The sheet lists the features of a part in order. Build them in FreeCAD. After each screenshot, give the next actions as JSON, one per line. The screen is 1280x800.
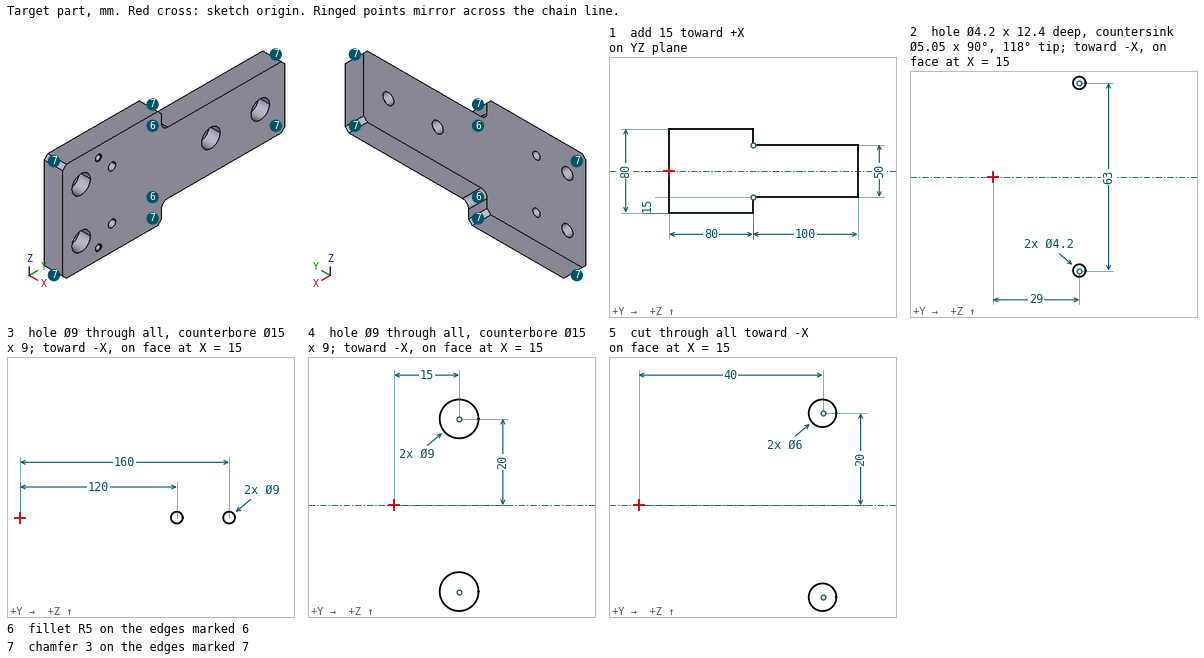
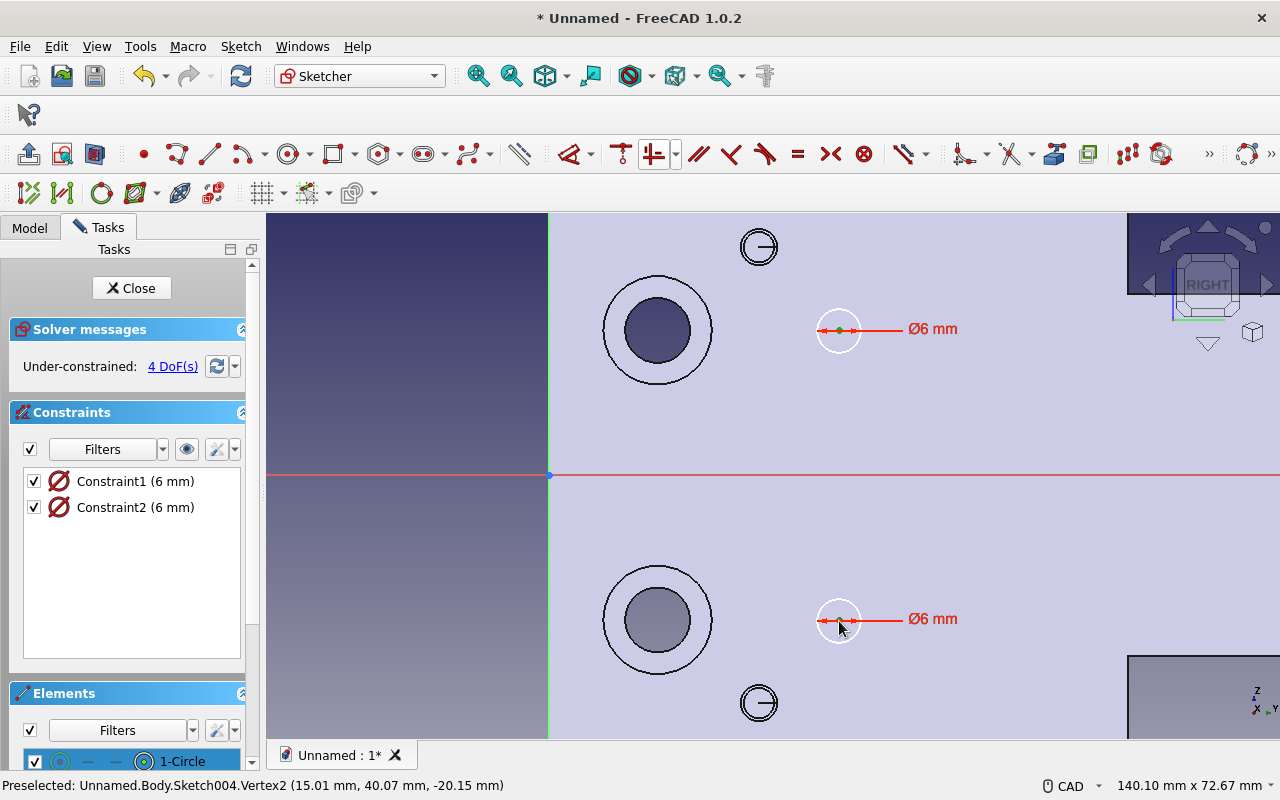
{"action": "left_click", "coordinate": [353, 475]}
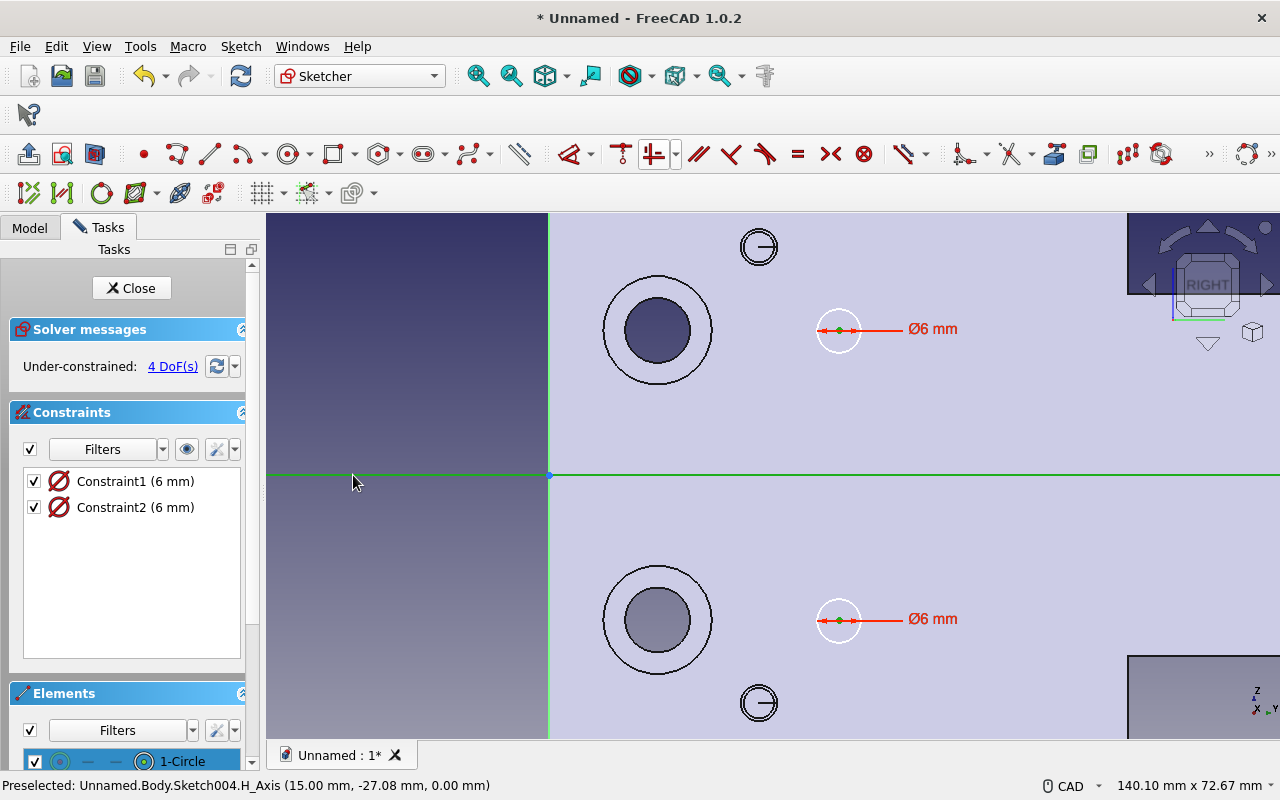
{"action": "left_click", "coordinate": [831, 154]}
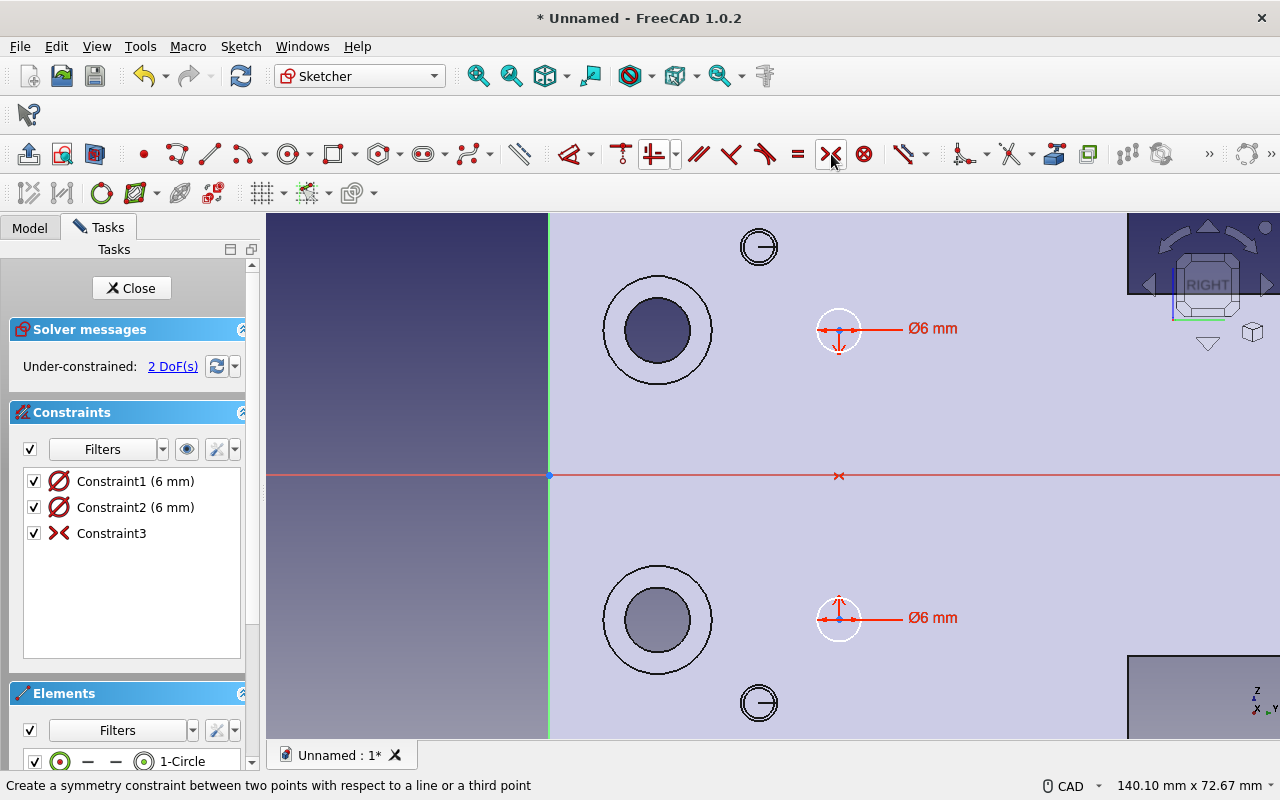
{"action": "key", "text": "d"}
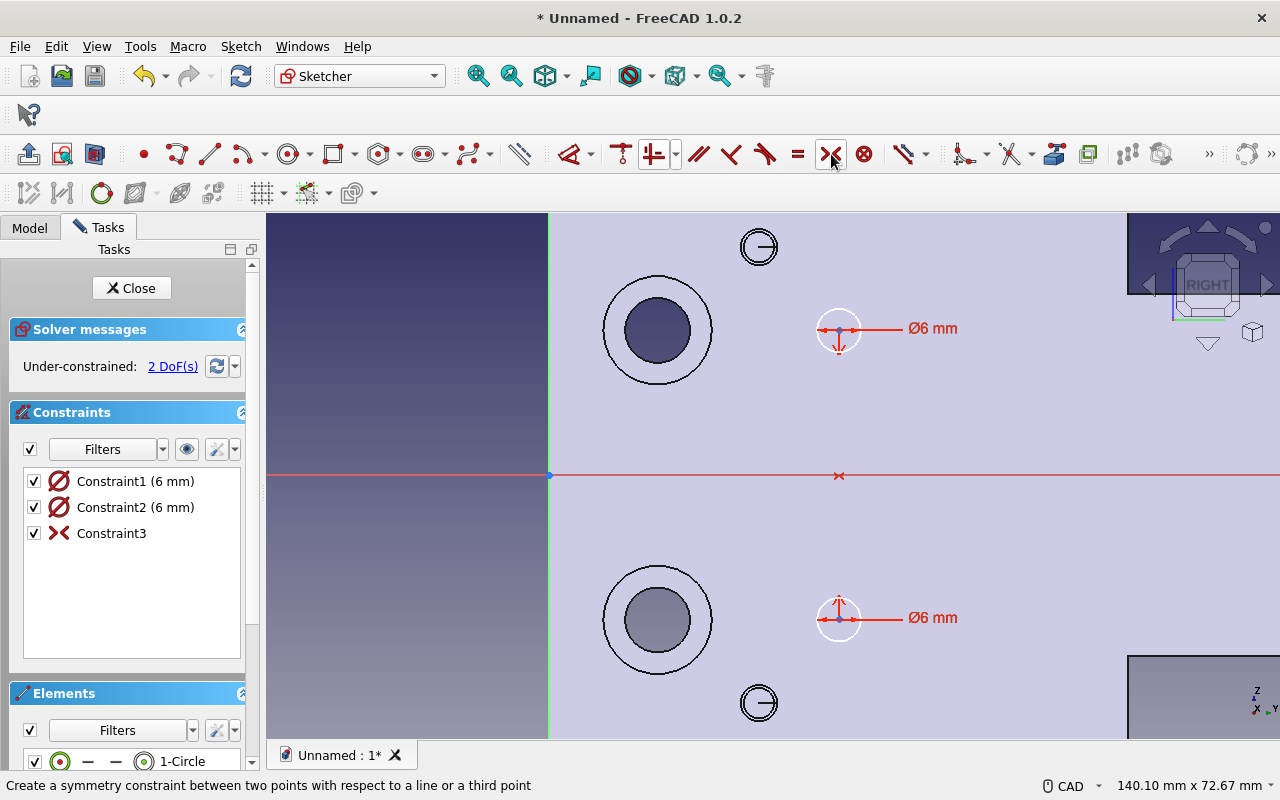
{"action": "left_click", "coordinate": [839, 330]}
{"action": "left_click", "coordinate": [694, 296]}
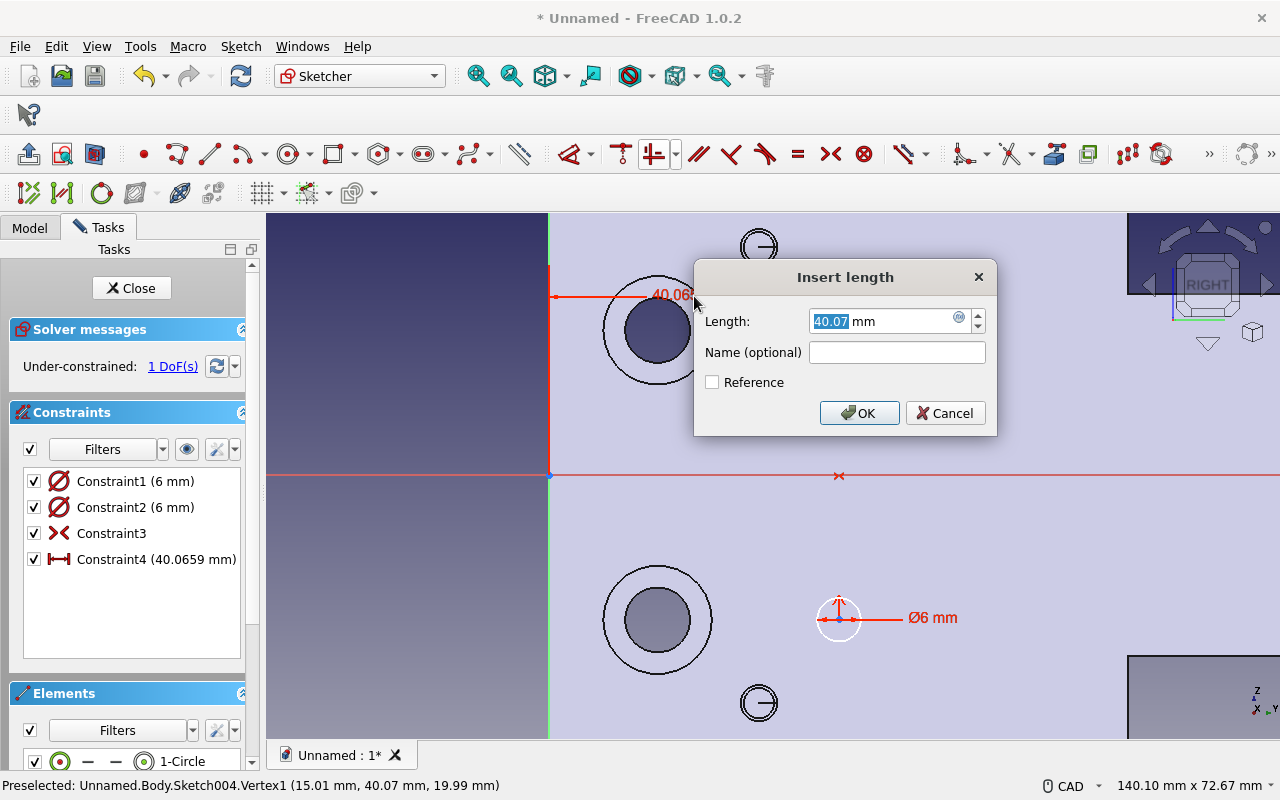
{"action": "type", "text": "40"}
{"action": "key", "text": "Return"}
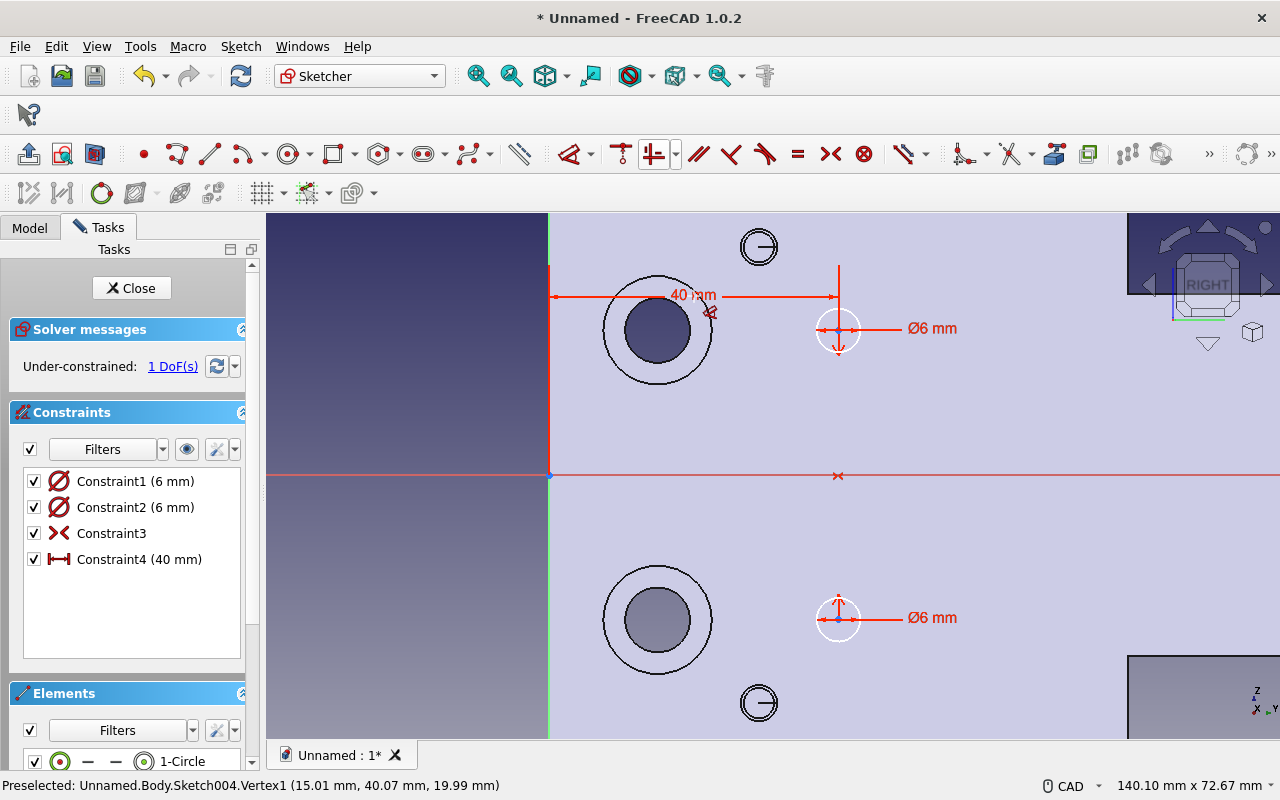
{"action": "left_click", "coordinate": [839, 330]}
{"action": "left_click", "coordinate": [515, 403]}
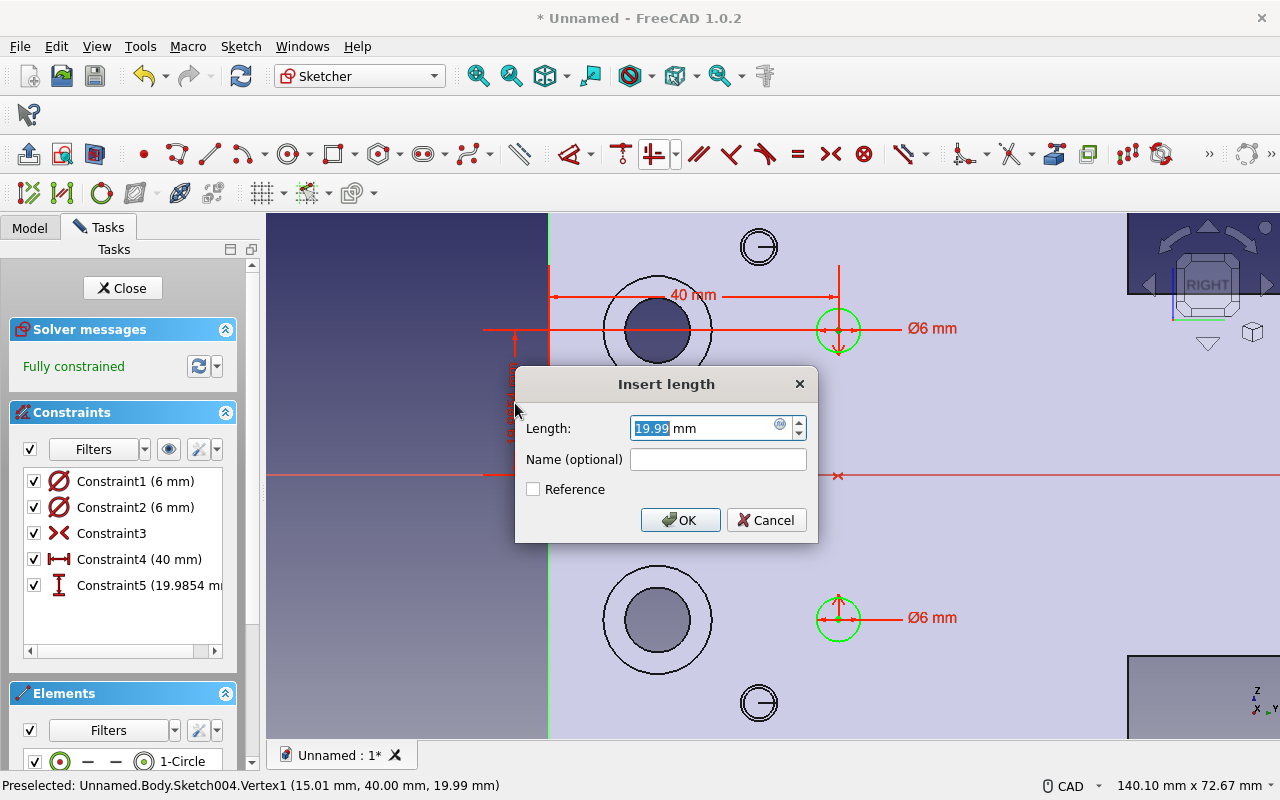
{"action": "type", "text": "20"}
{"action": "key", "text": "Return"}
{"action": "key", "text": "Escape"}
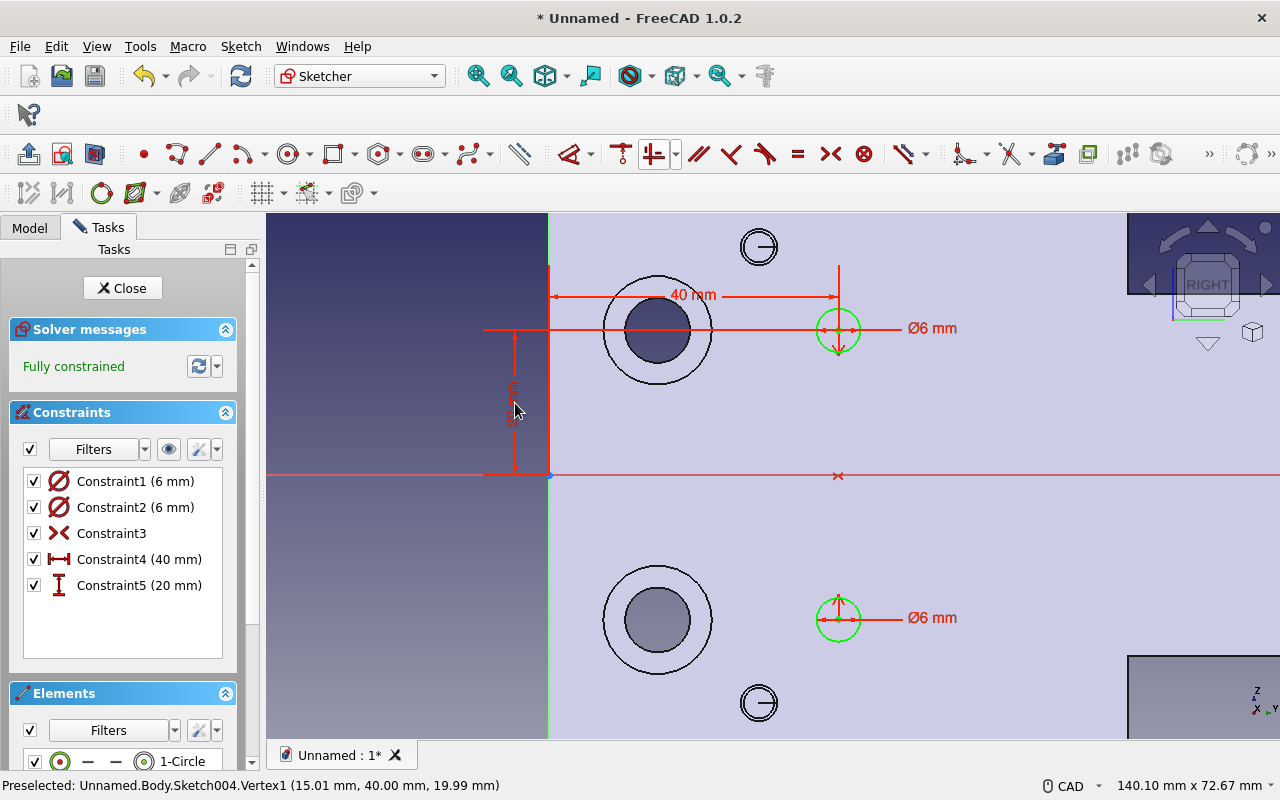
{"action": "left_click", "coordinate": [123, 288]}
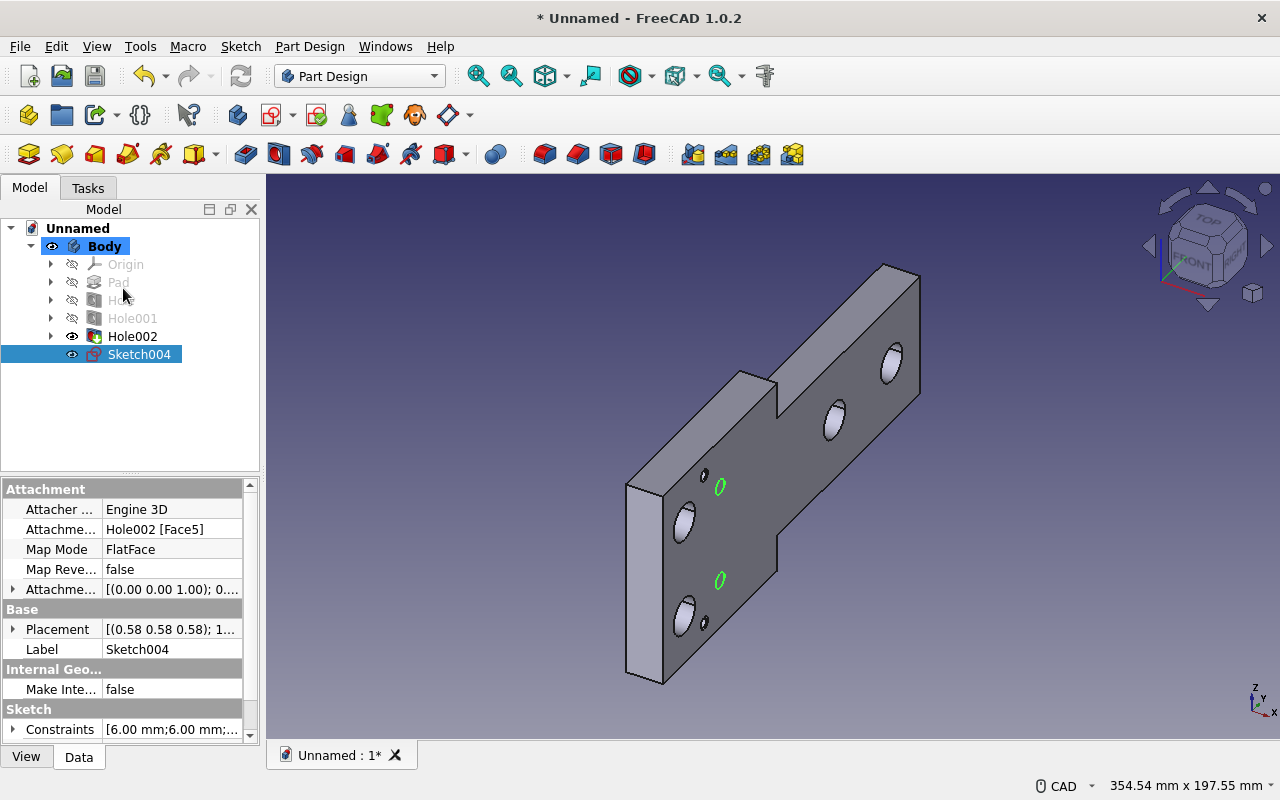
{"action": "left_click", "coordinate": [246, 154]}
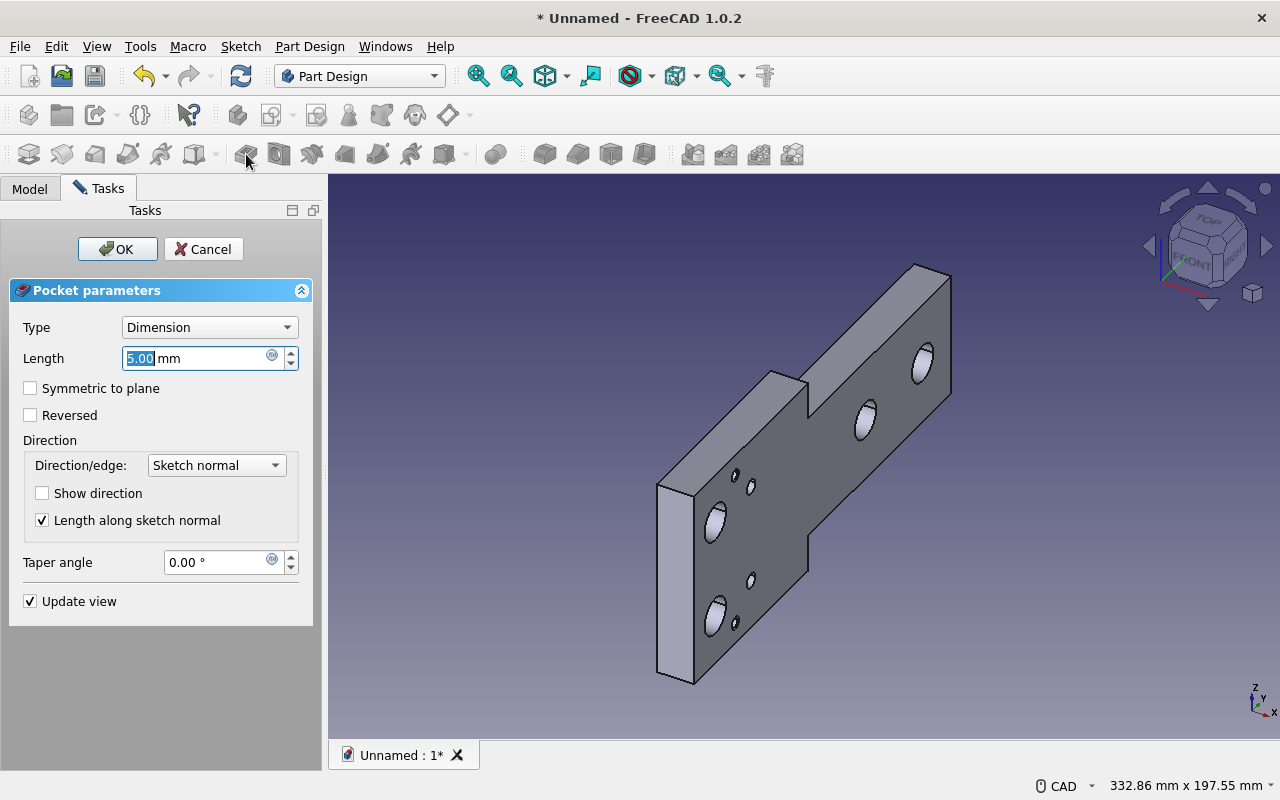
{"action": "left_click", "coordinate": [210, 328]}